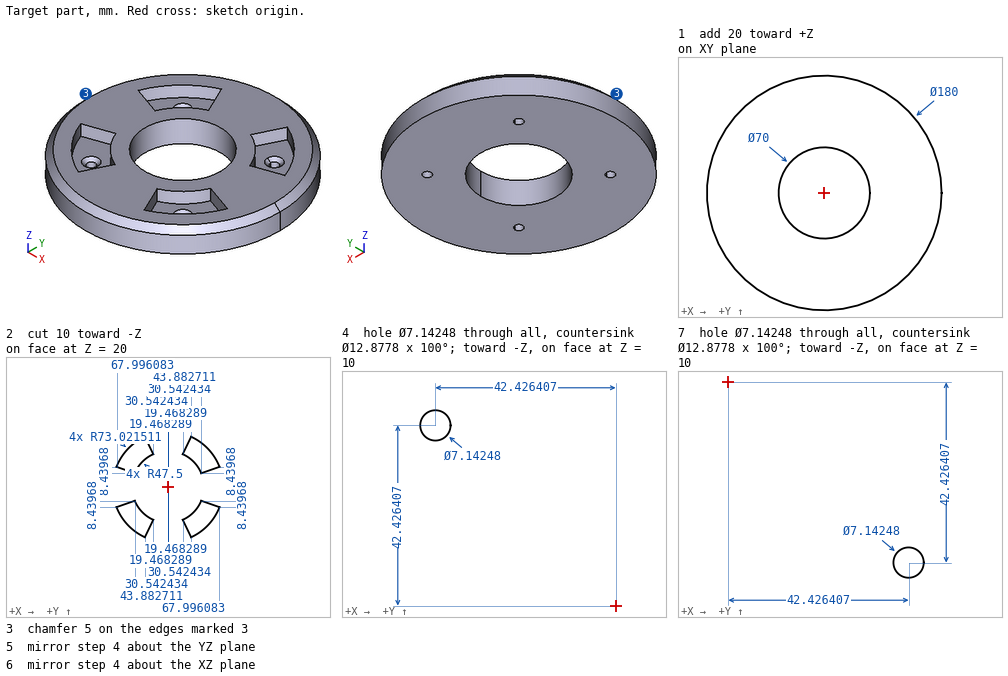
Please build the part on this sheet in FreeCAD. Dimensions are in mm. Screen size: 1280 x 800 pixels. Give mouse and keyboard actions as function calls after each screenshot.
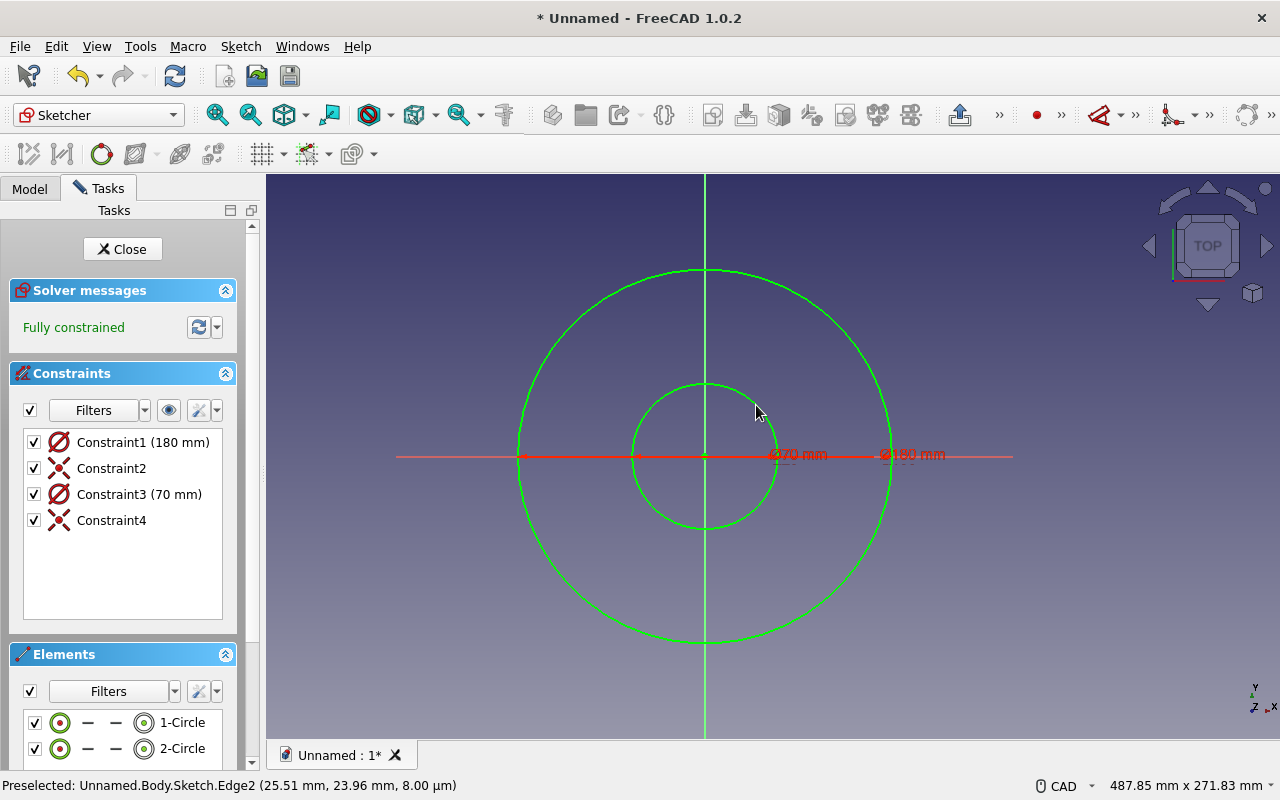
click(123, 249)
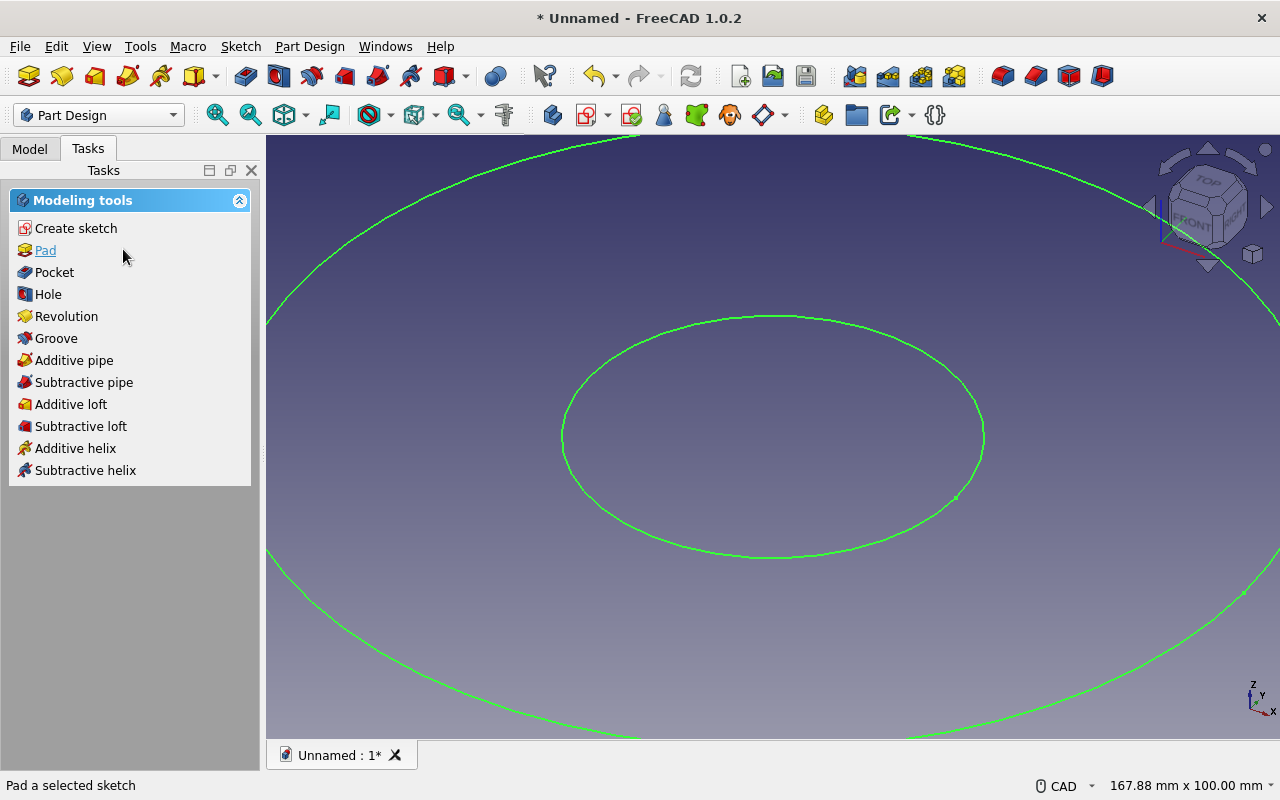
click(29, 76)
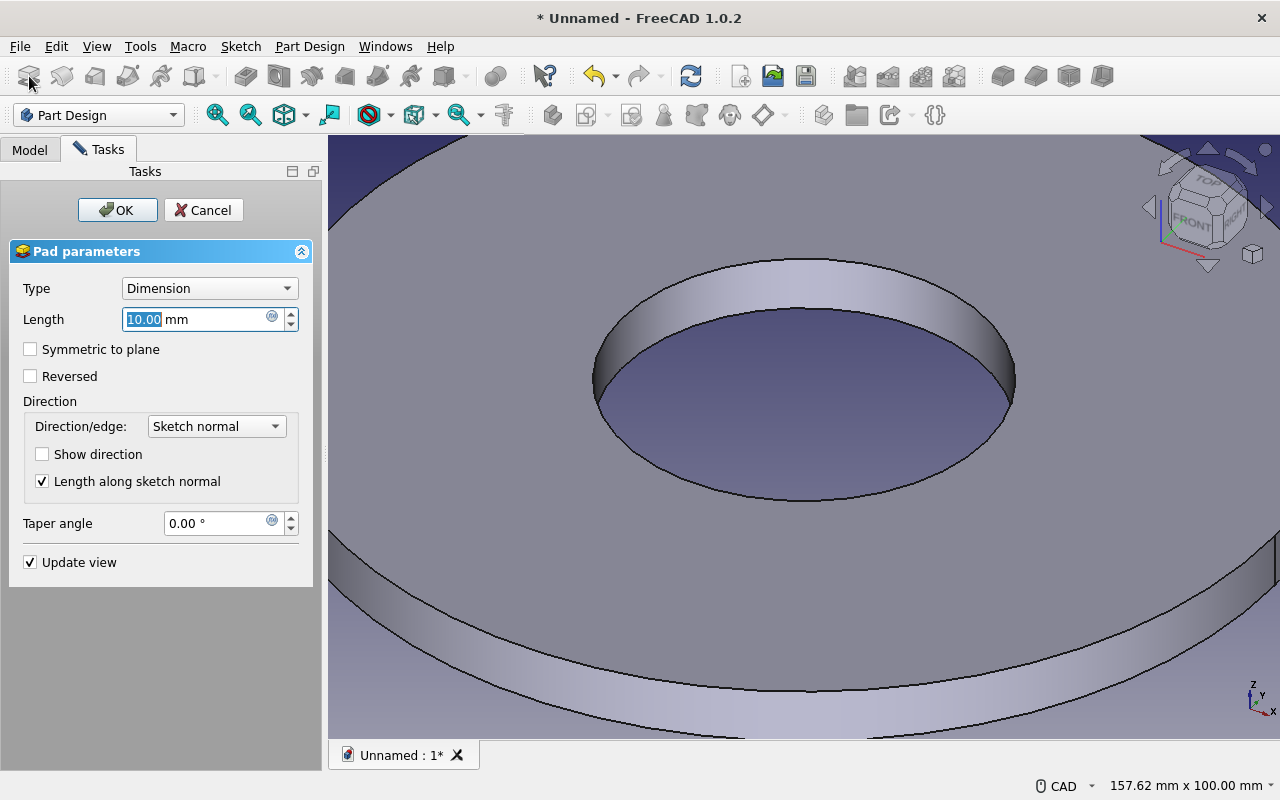
text(20)
key(Tab)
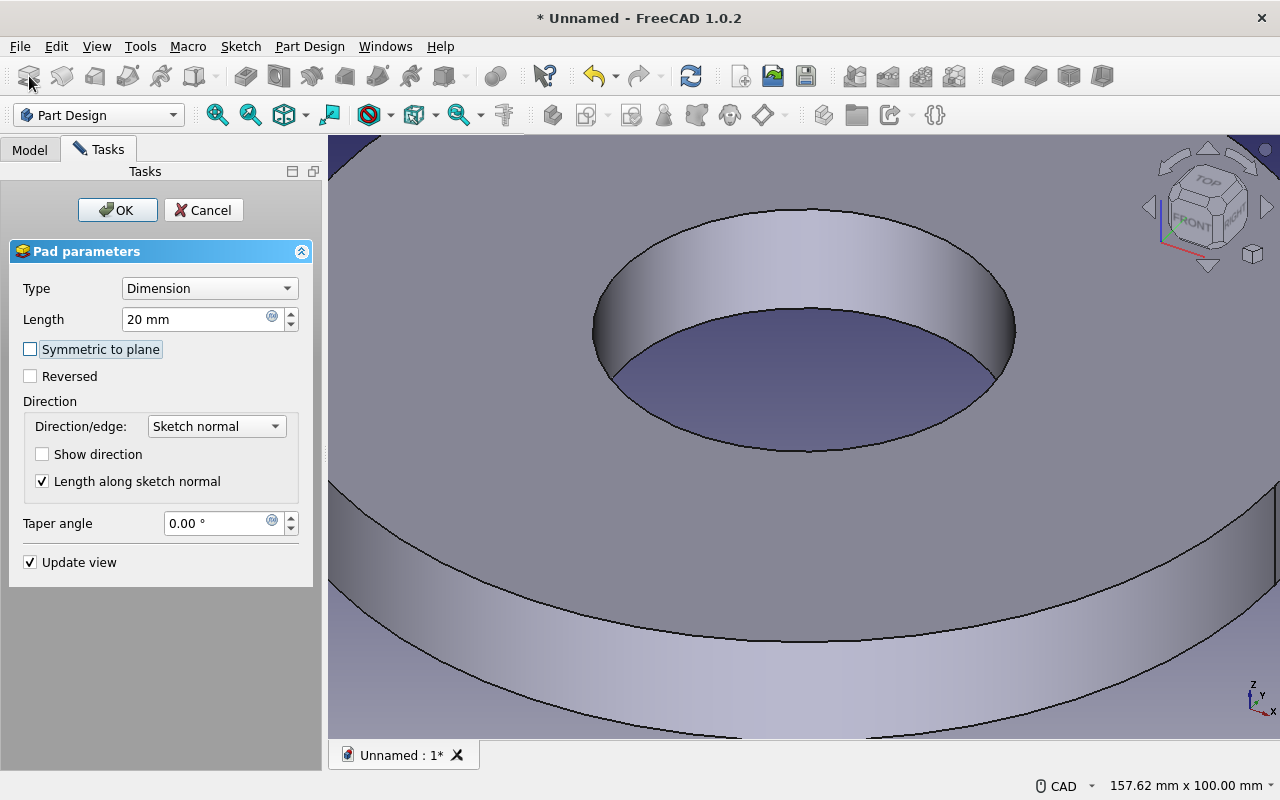
click(118, 210)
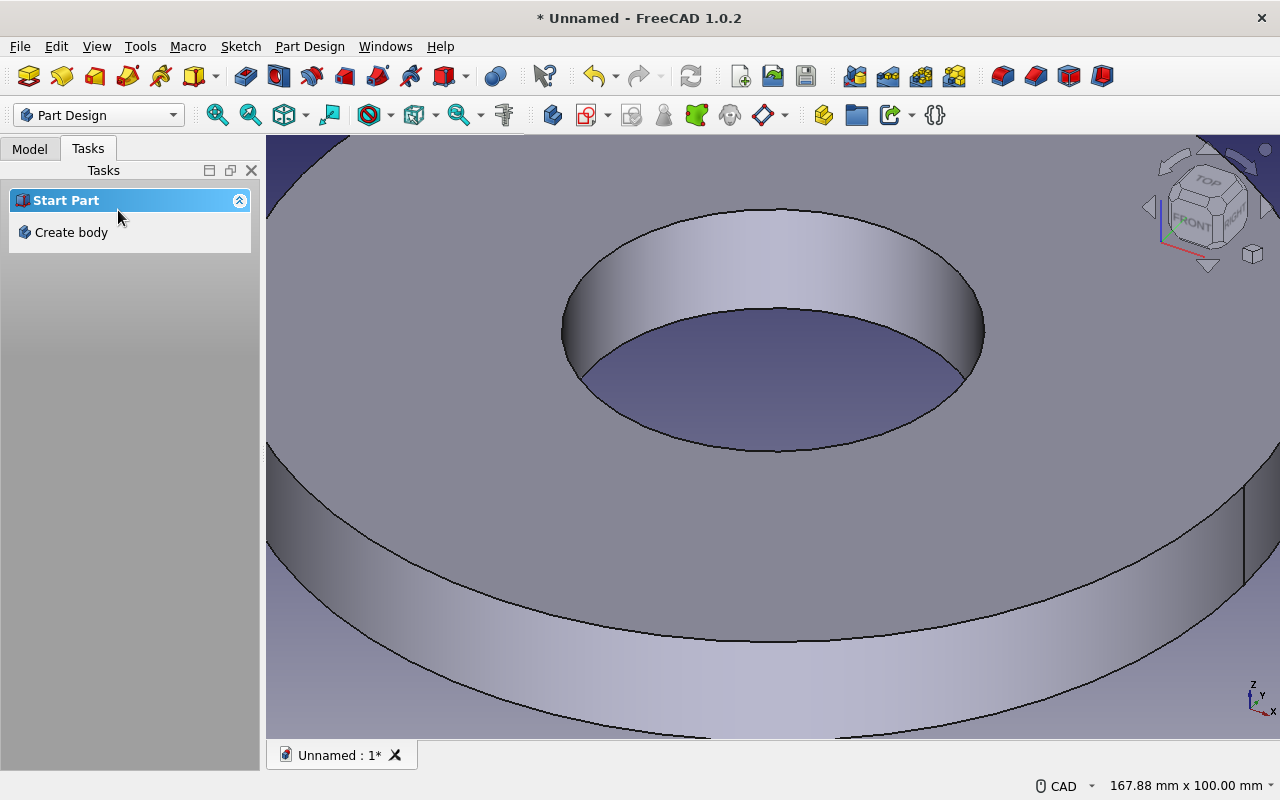
click(218, 116)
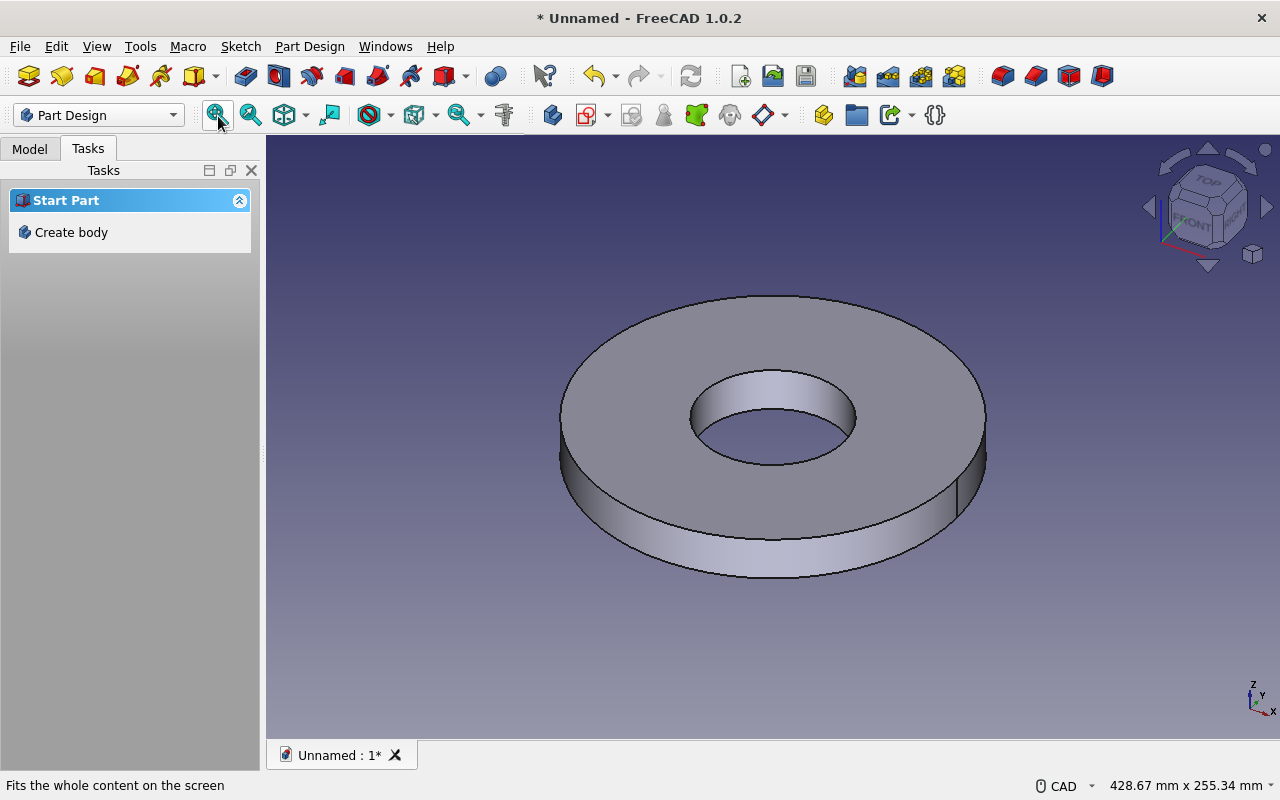
click(659, 460)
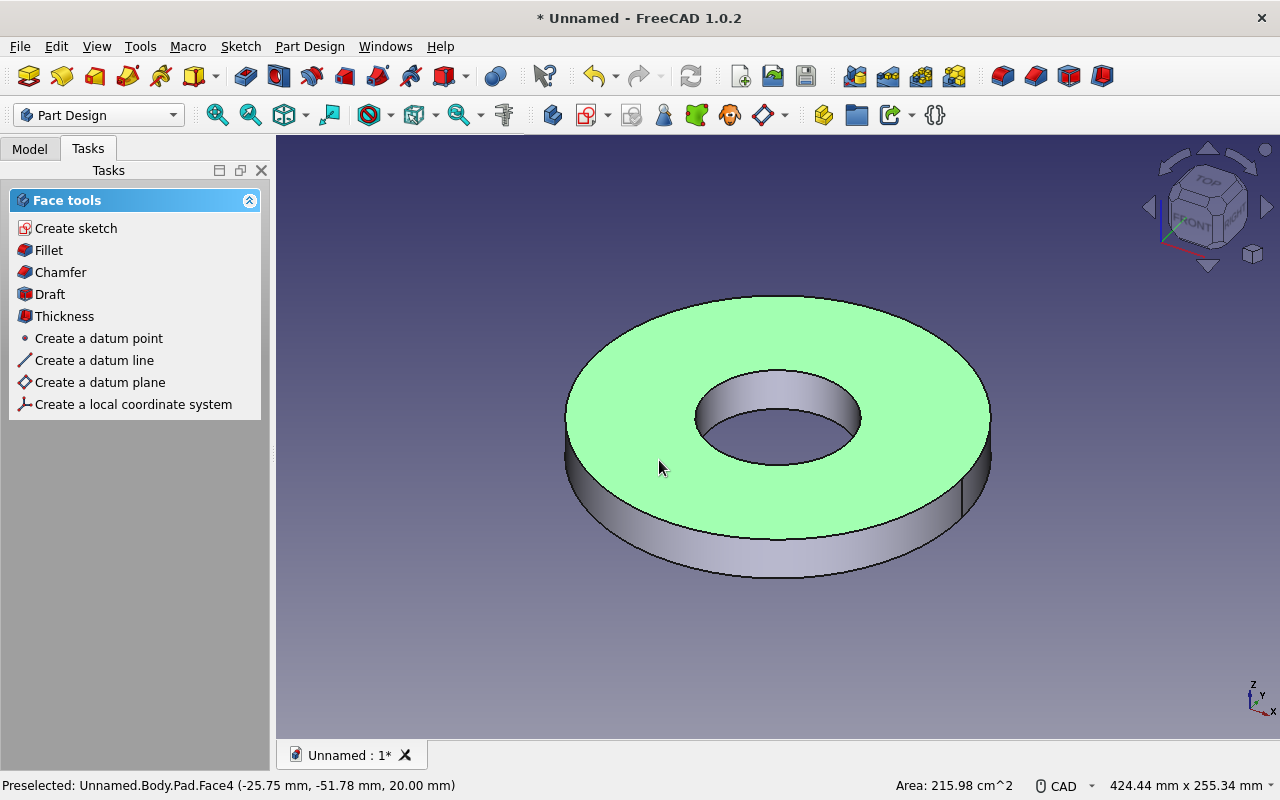
click(586, 116)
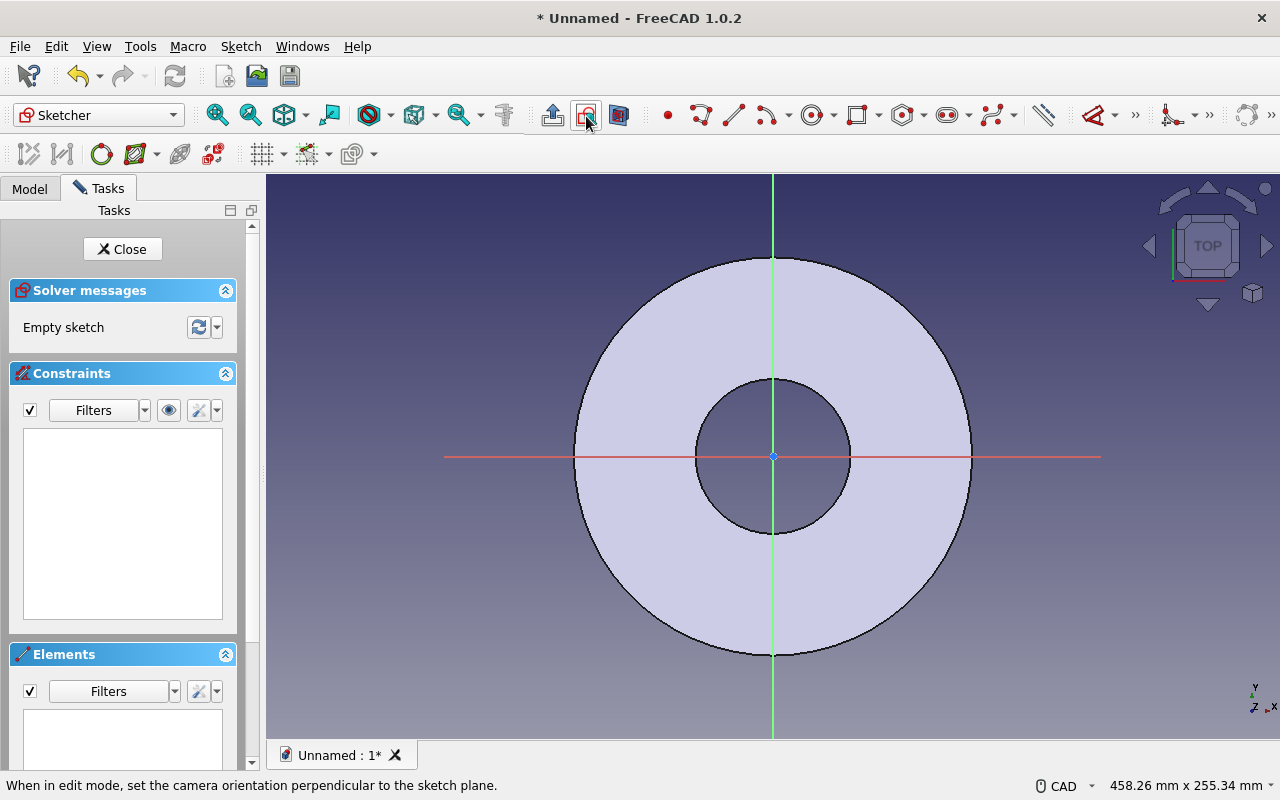
click(734, 116)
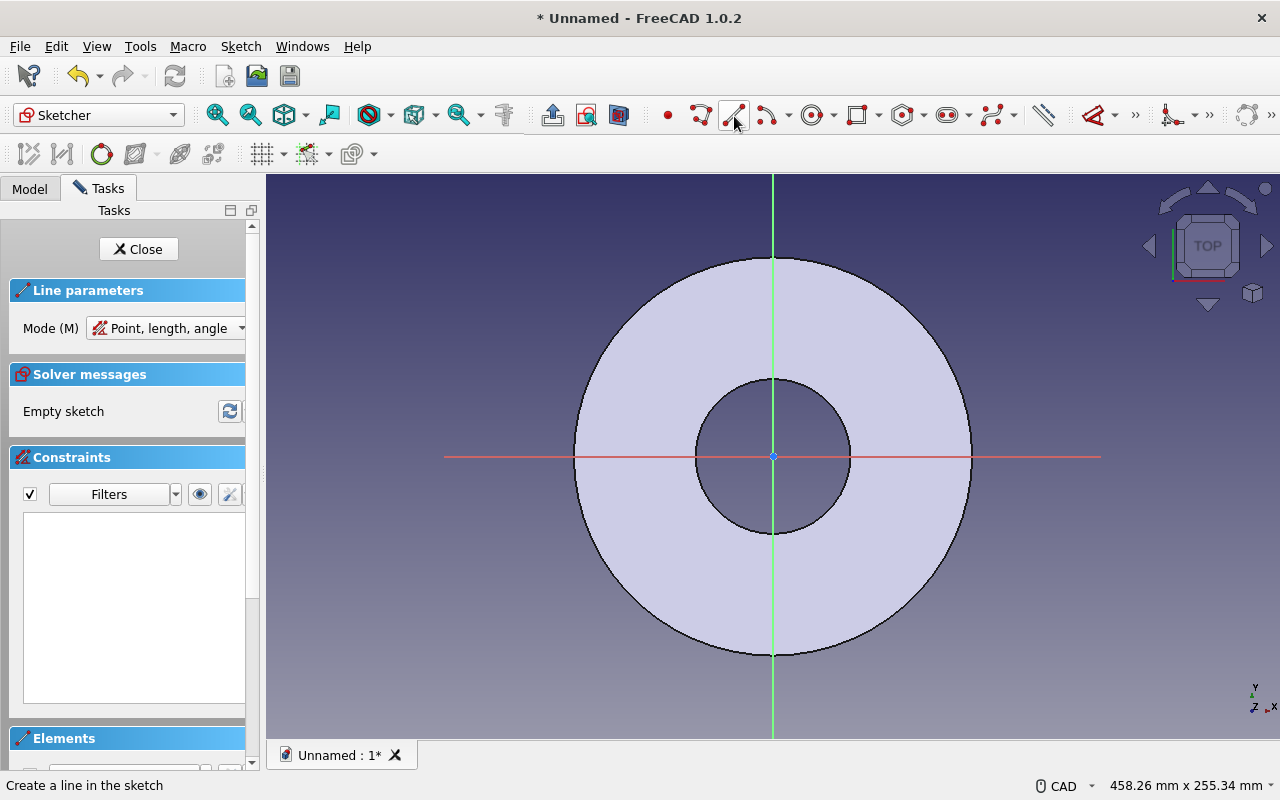
click(730, 361)
click(705, 310)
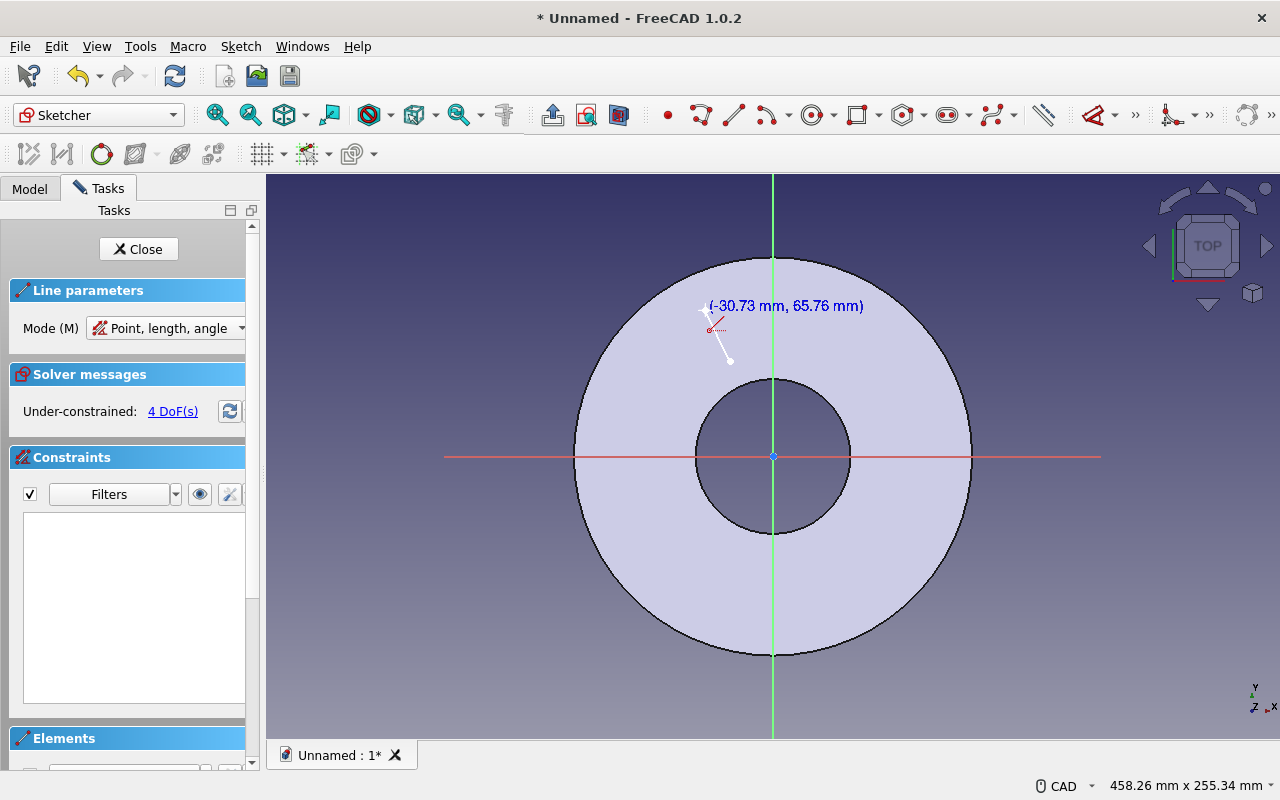
click(623, 398)
click(676, 416)